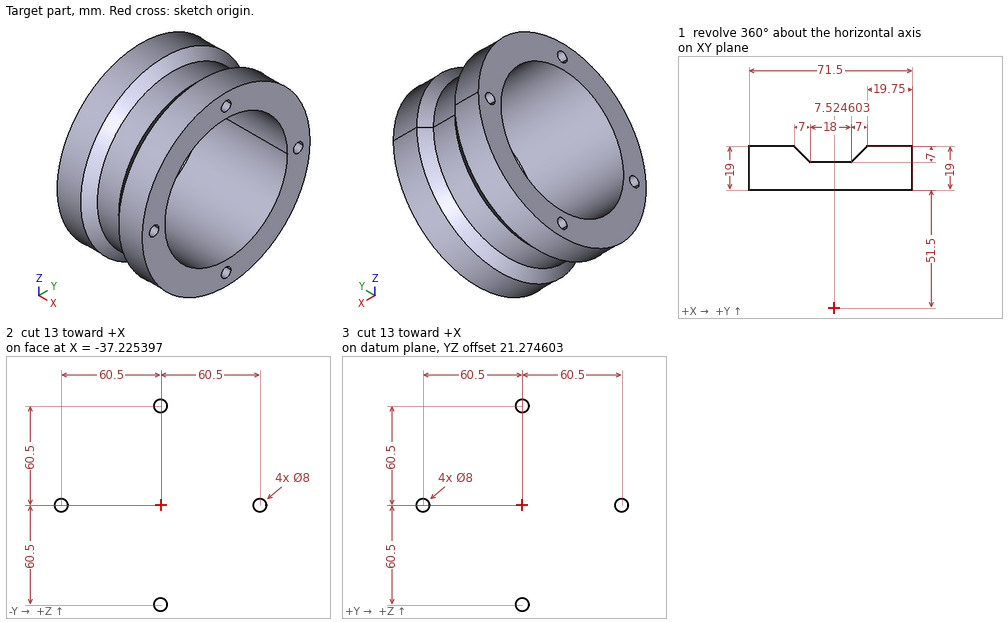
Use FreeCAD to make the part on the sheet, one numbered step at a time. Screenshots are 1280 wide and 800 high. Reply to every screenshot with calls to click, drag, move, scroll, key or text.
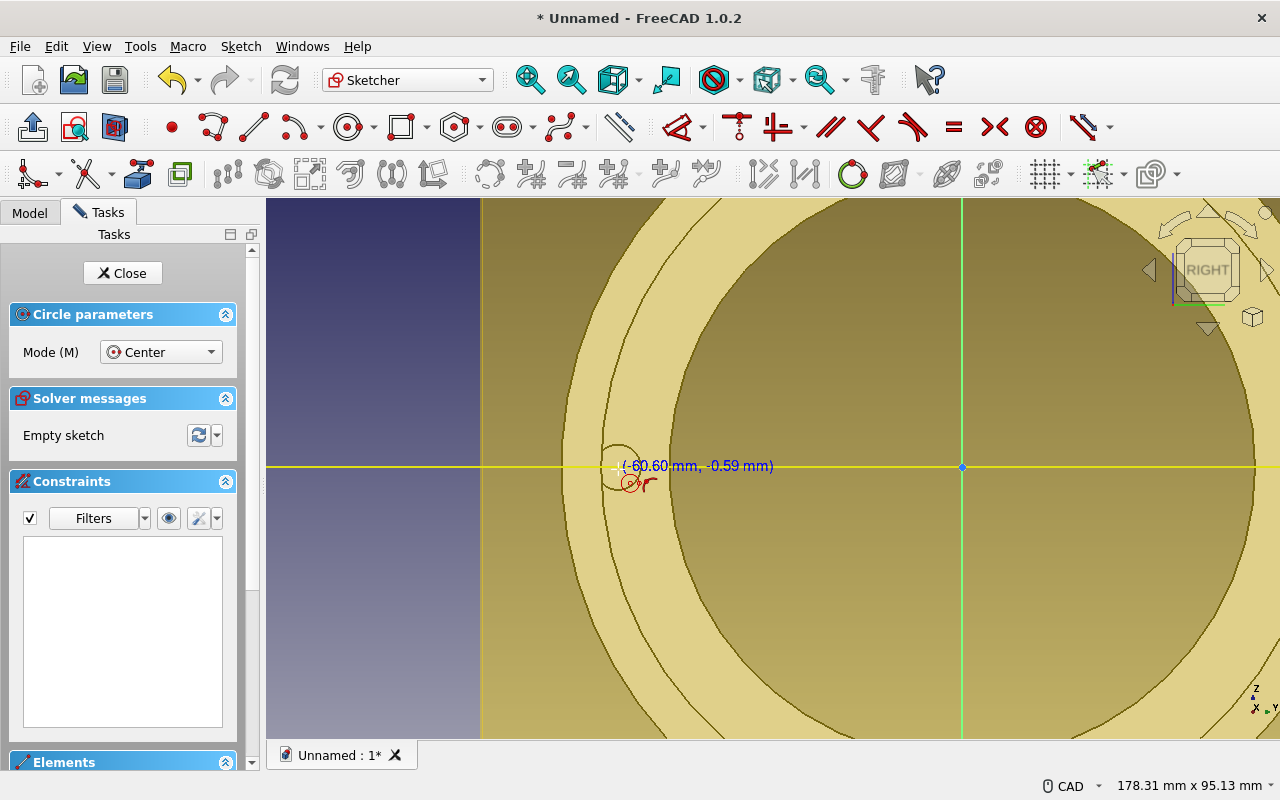
click(618, 467)
move(634, 451)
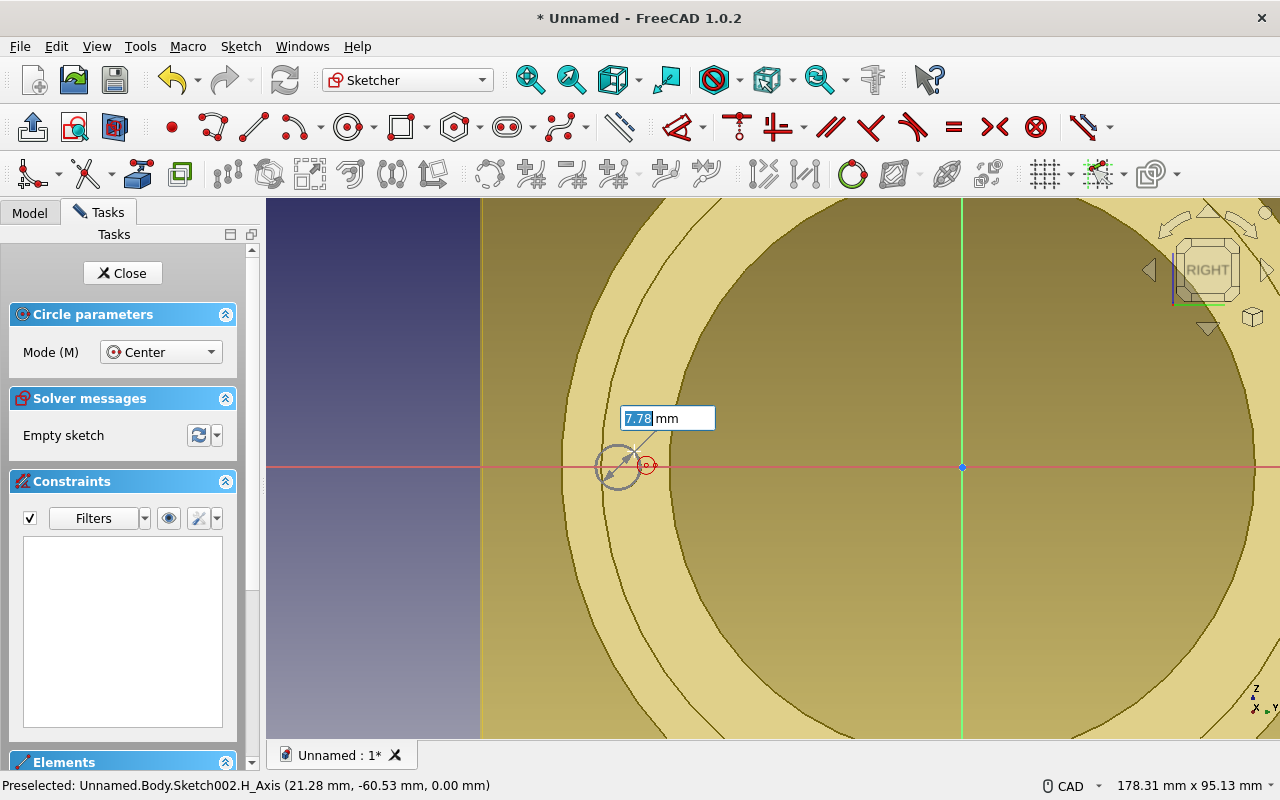
text(8)
key(Return)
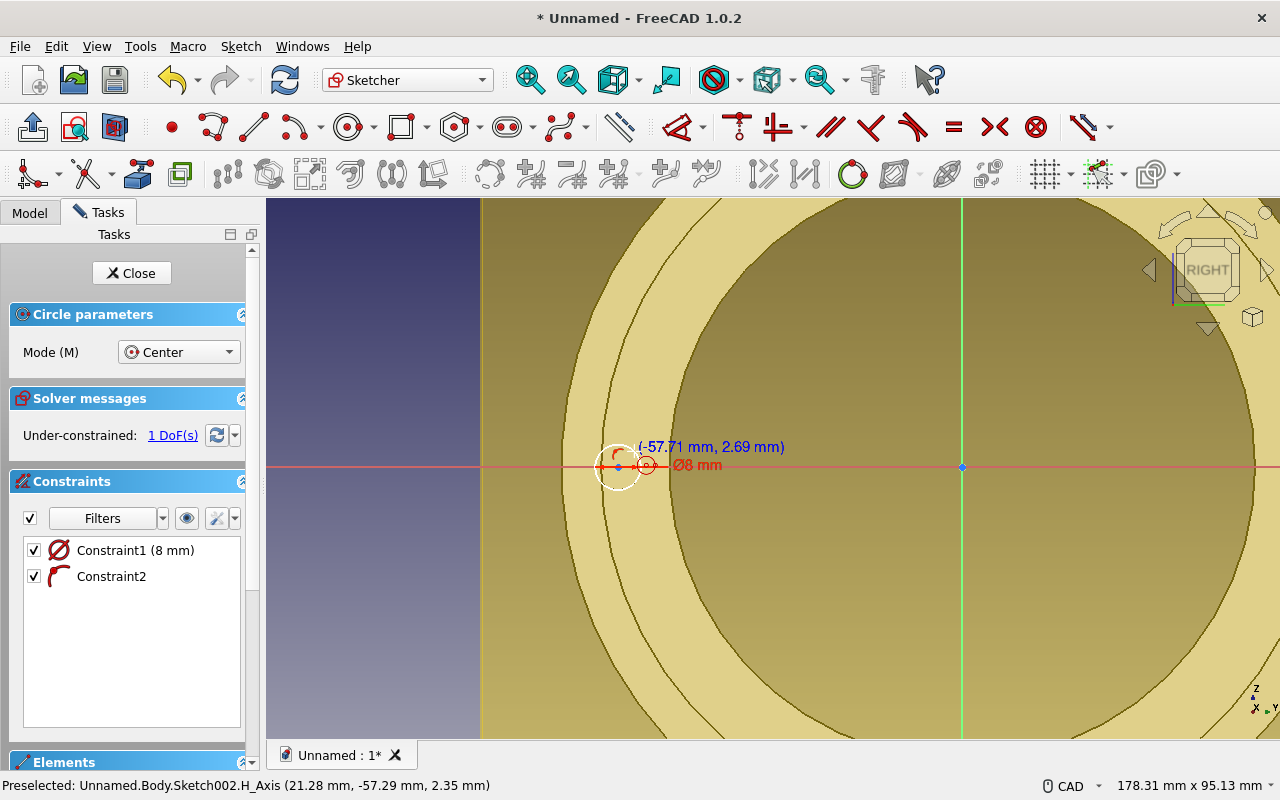
scroll(494, 470, down, 4)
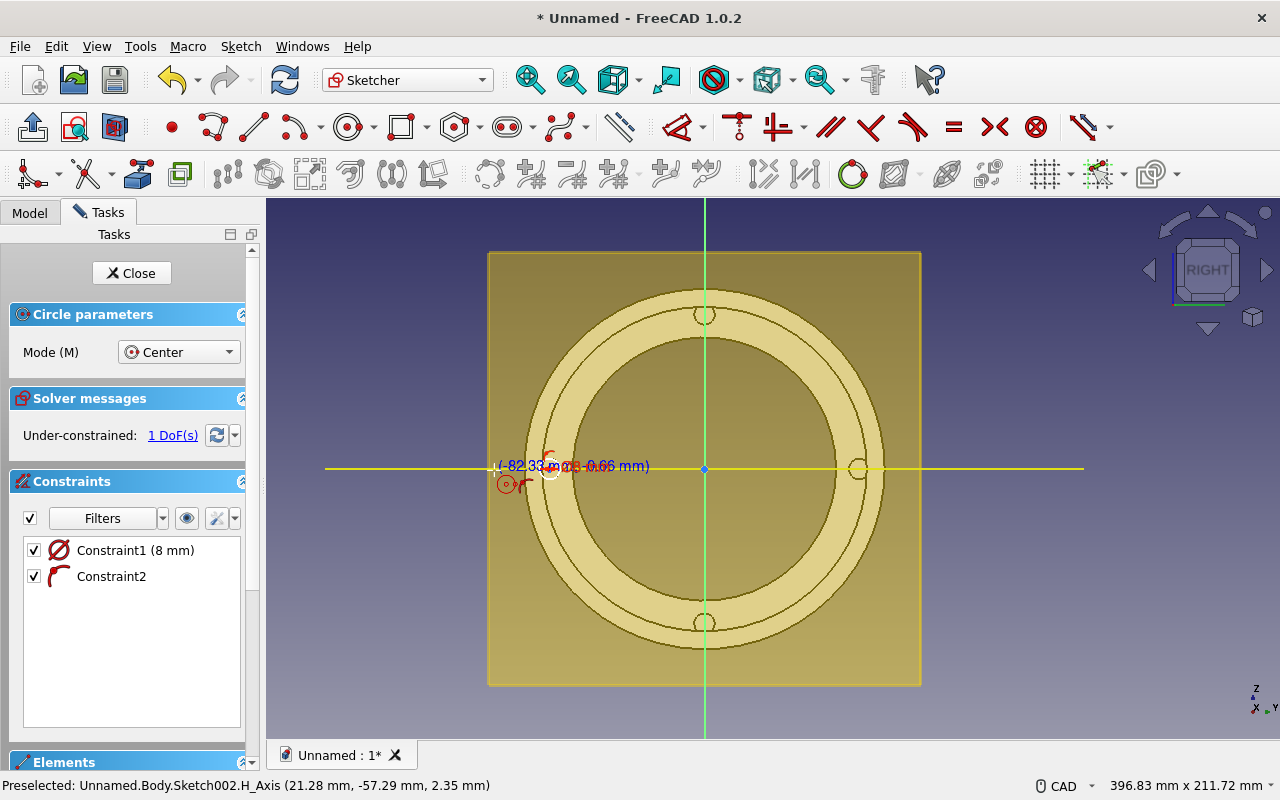
scroll(705, 314, up, 4)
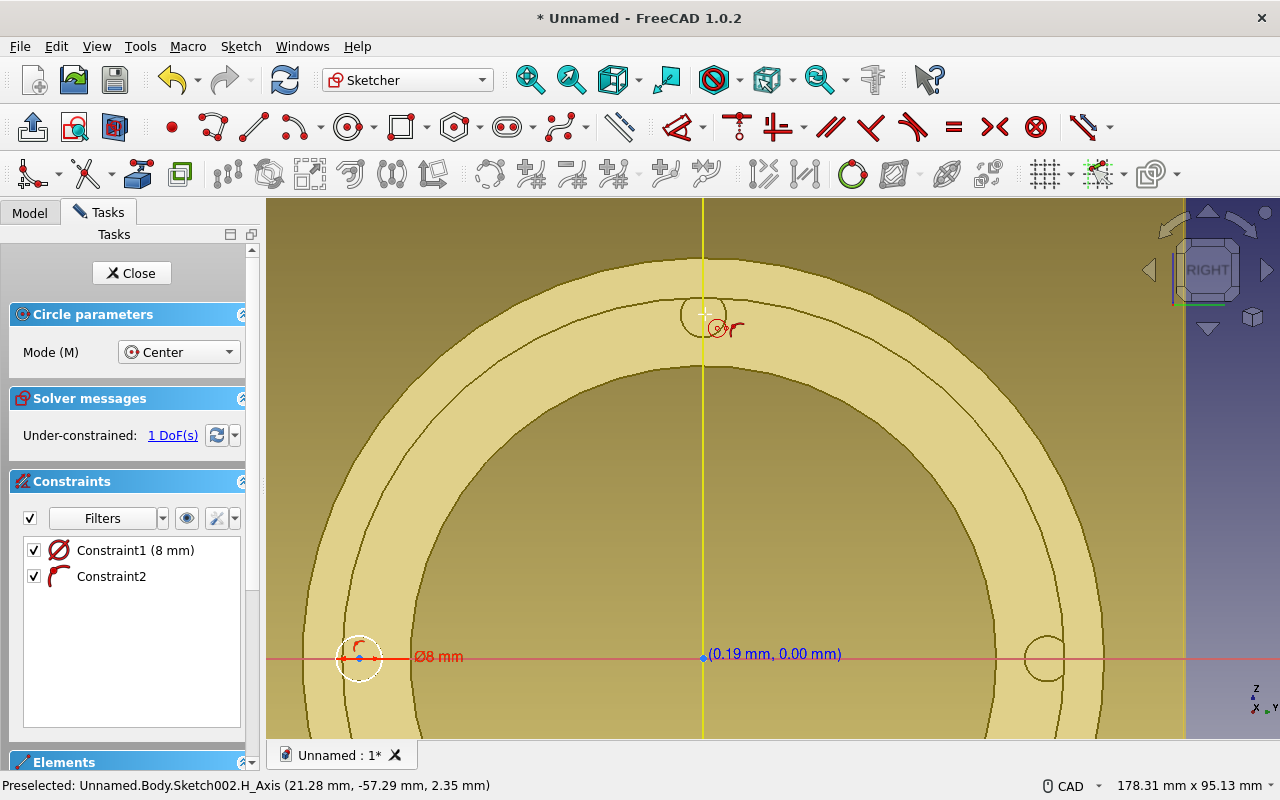
click(703, 315)
move(719, 299)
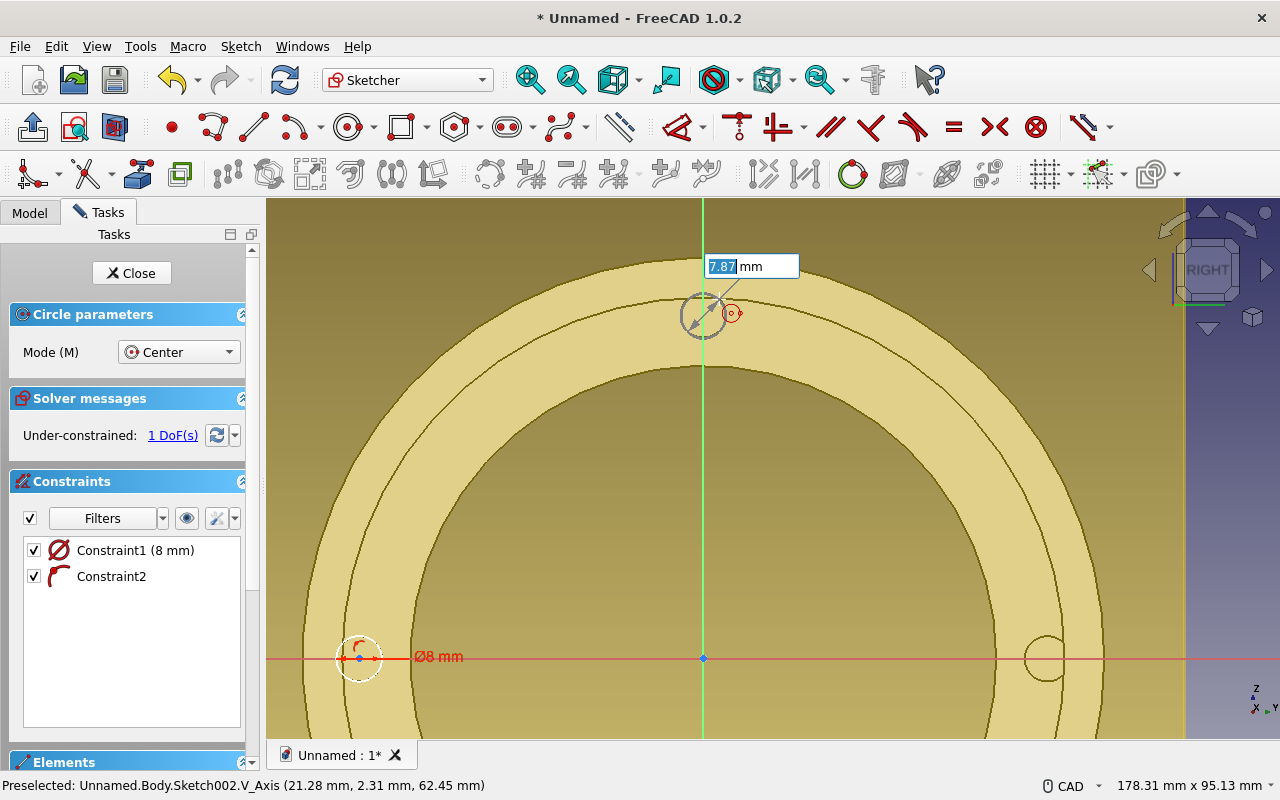
text(8)
key(Return)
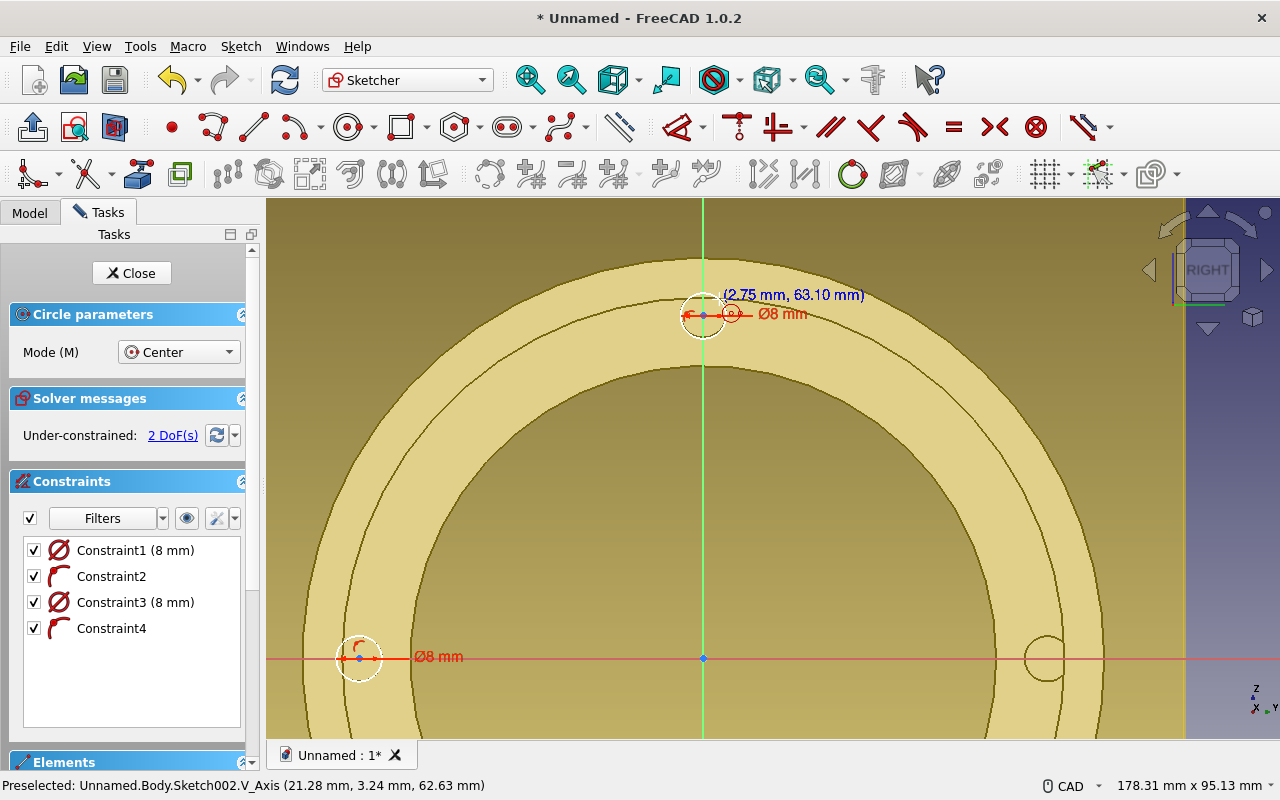
click(1047, 659)
move(1063, 643)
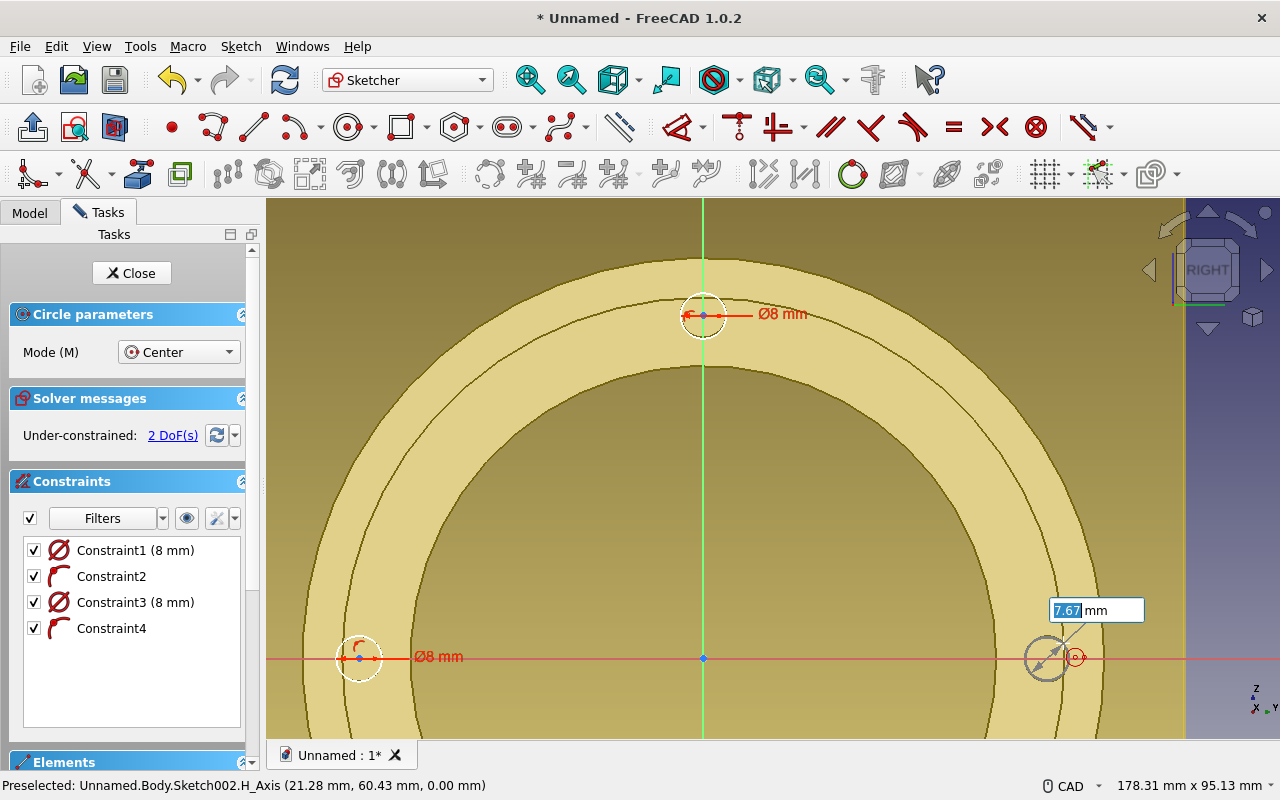
text(8)
key(Return)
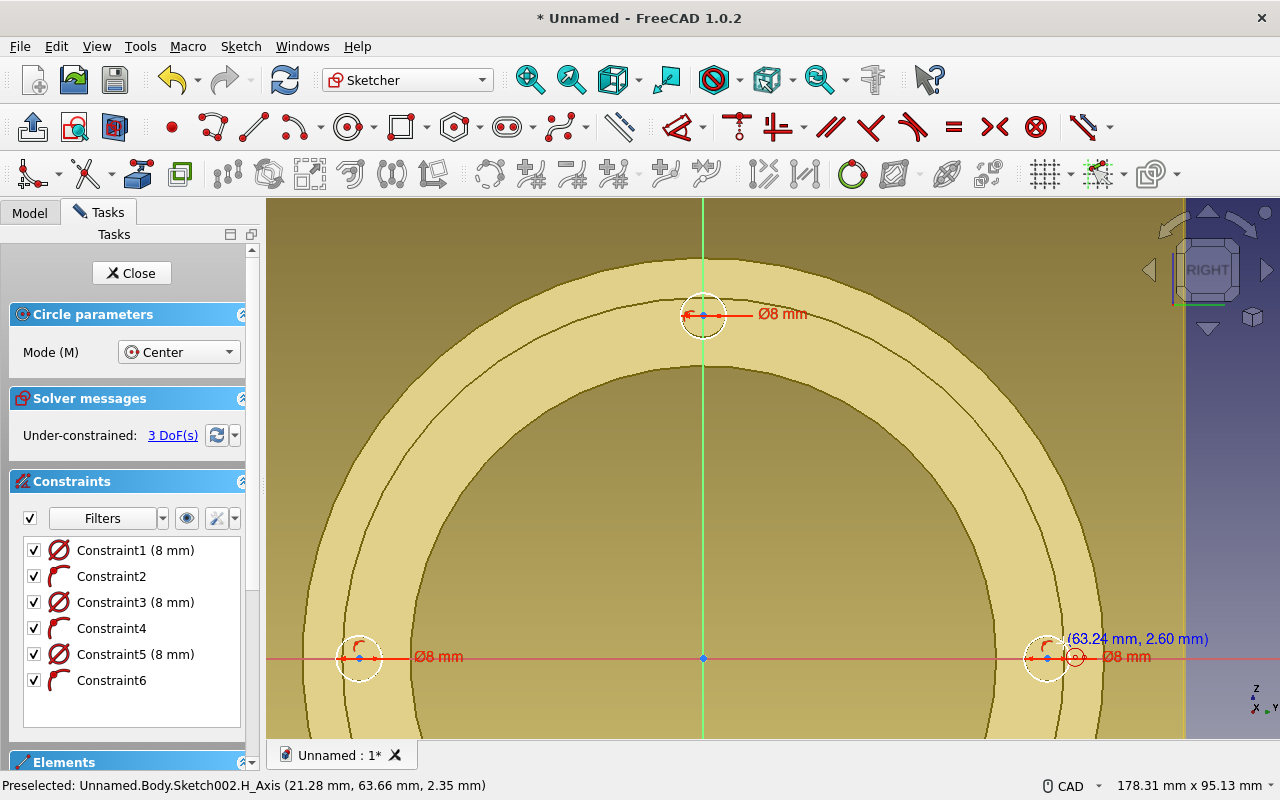
scroll(705, 313, down, 4)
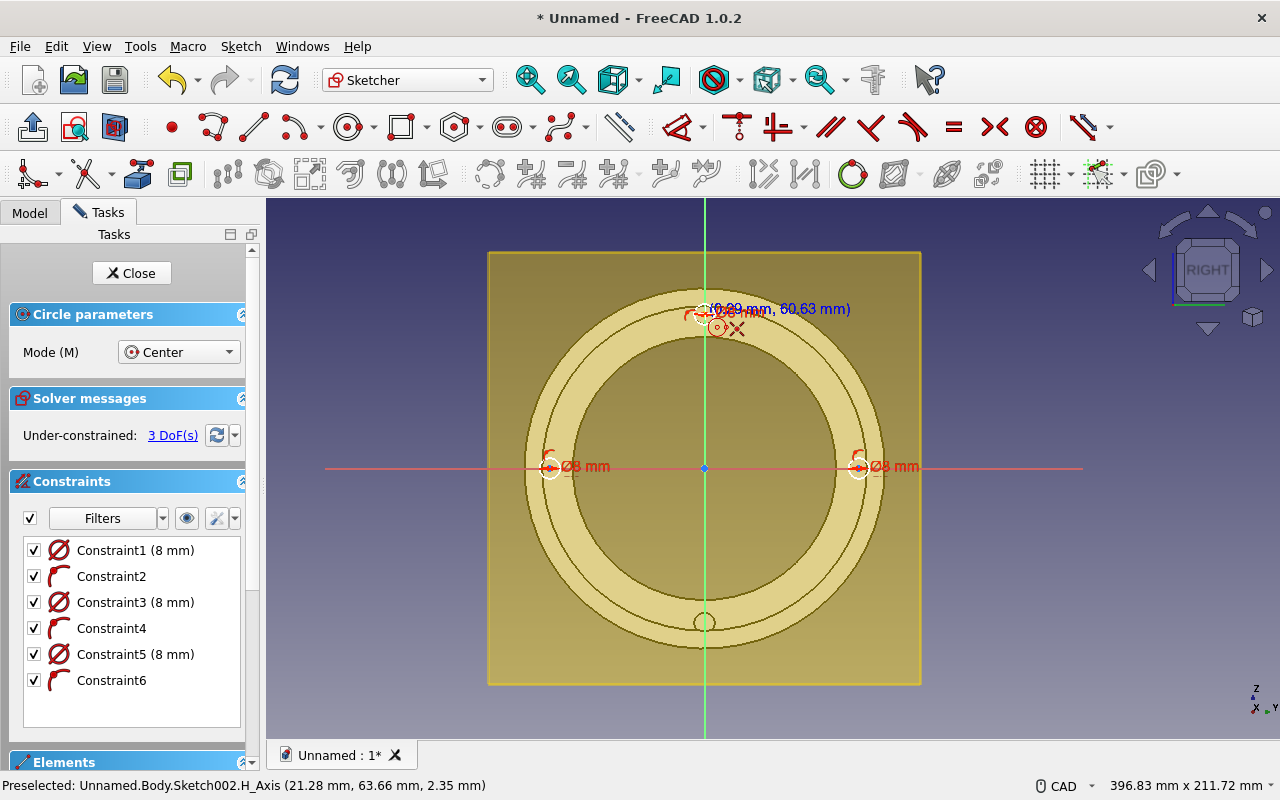
scroll(705, 623, up, 4)